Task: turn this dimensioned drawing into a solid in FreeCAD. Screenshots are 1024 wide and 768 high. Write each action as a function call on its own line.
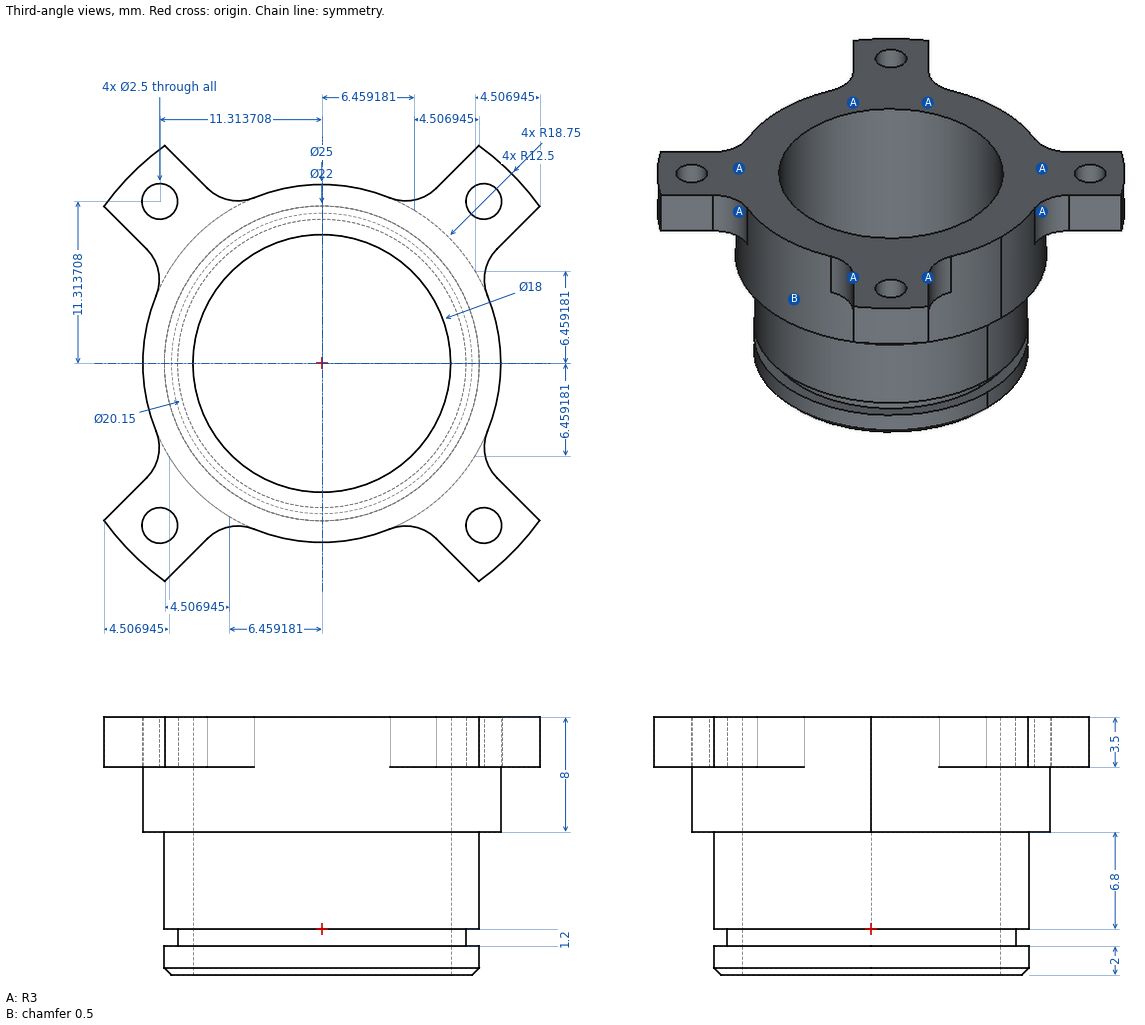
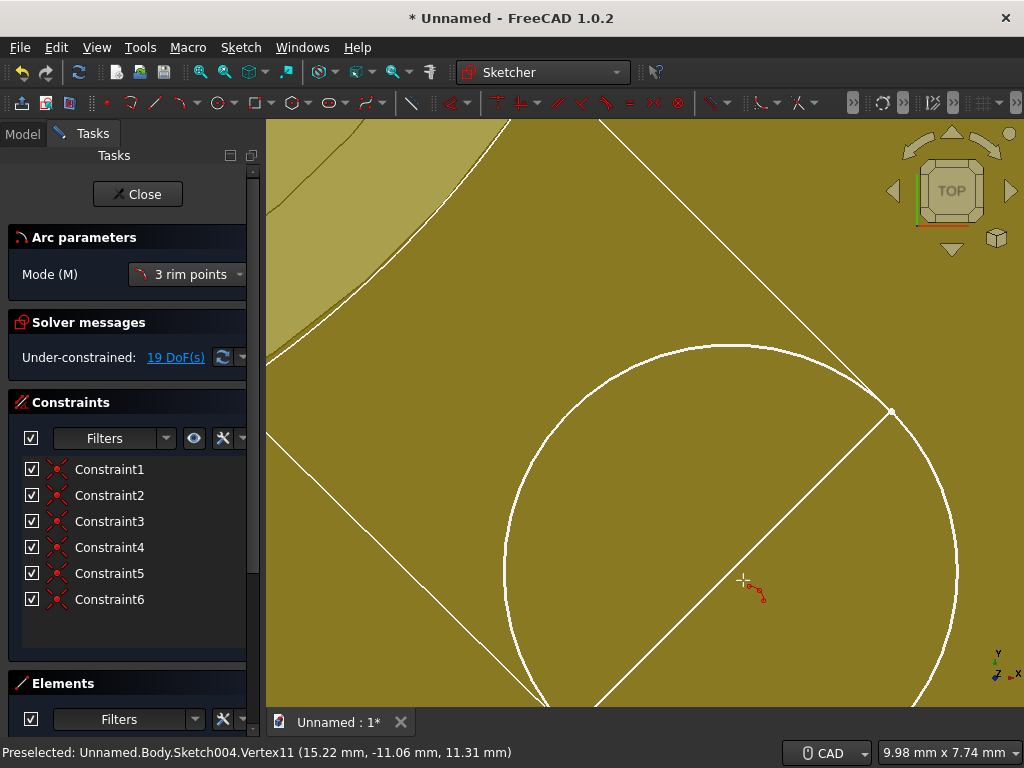
click(742, 578)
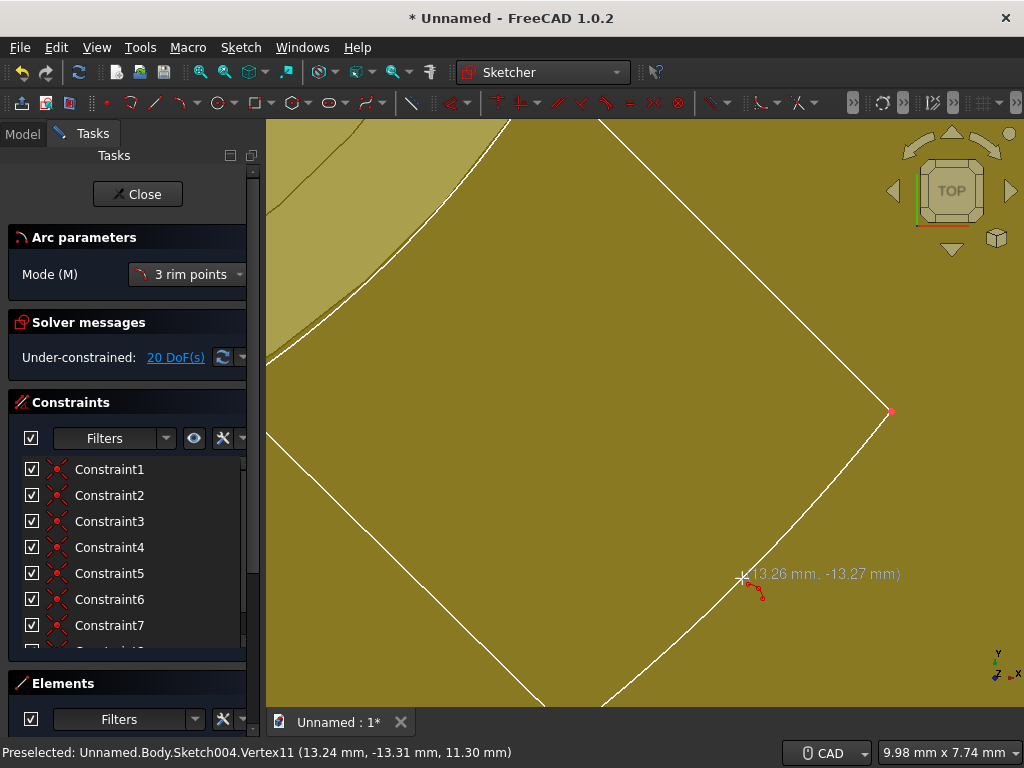
click(156, 104)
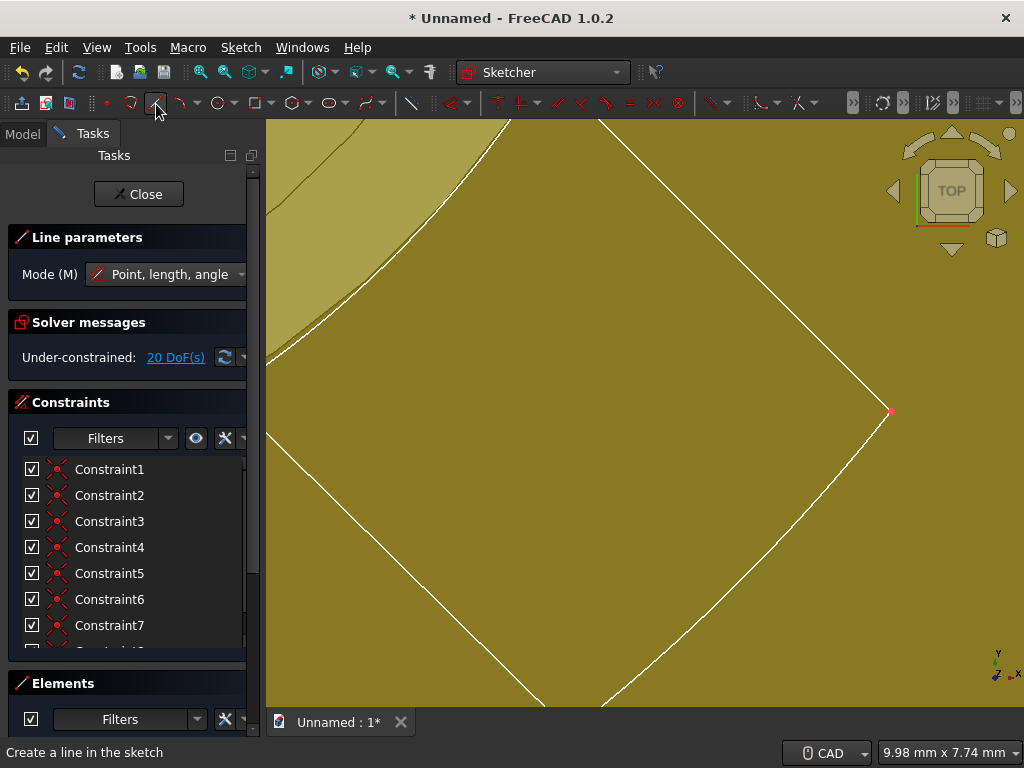
scroll(743, 580, down, 9)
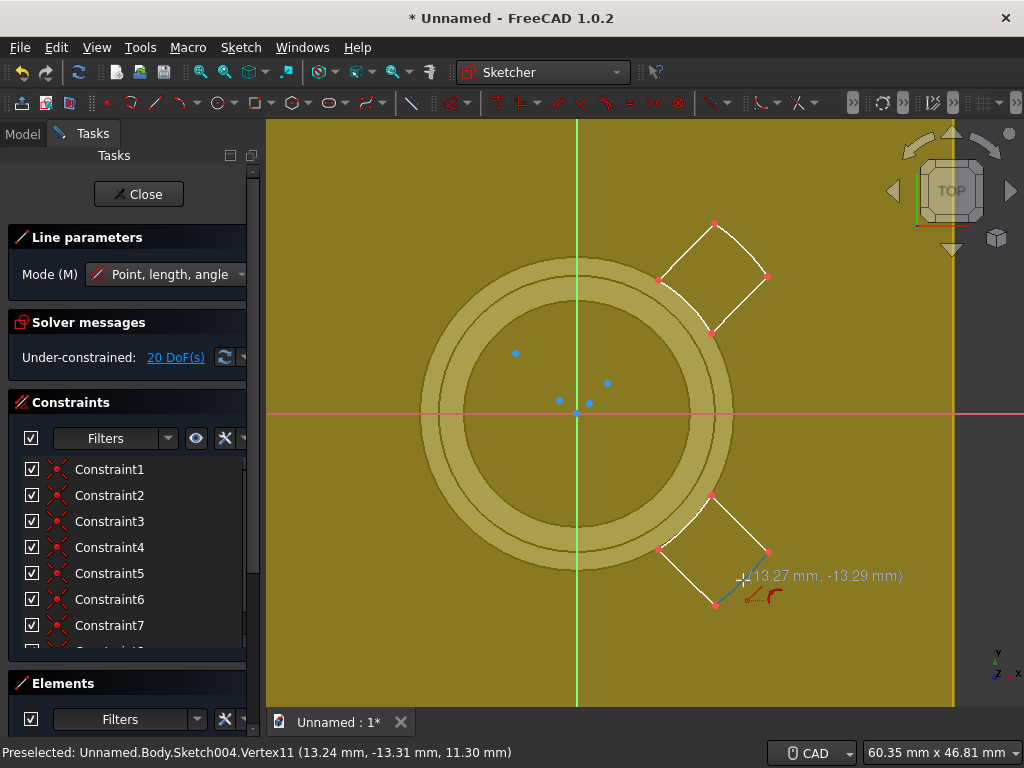
click(439, 605)
click(496, 548)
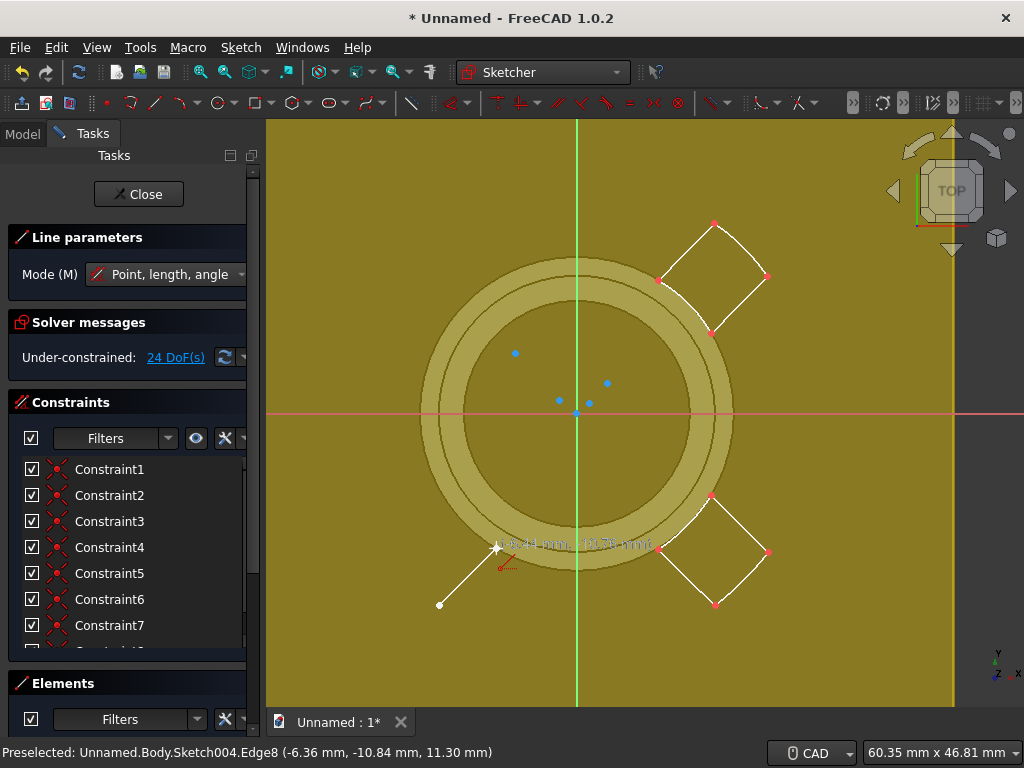
click(442, 495)
click(386, 552)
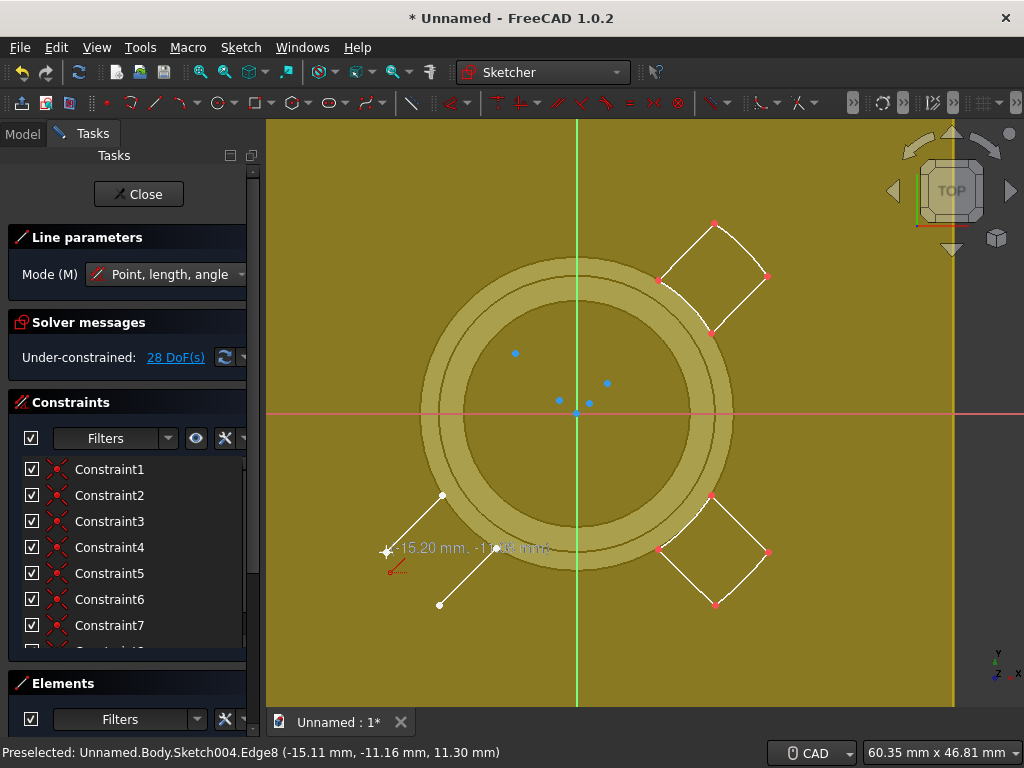
click(180, 104)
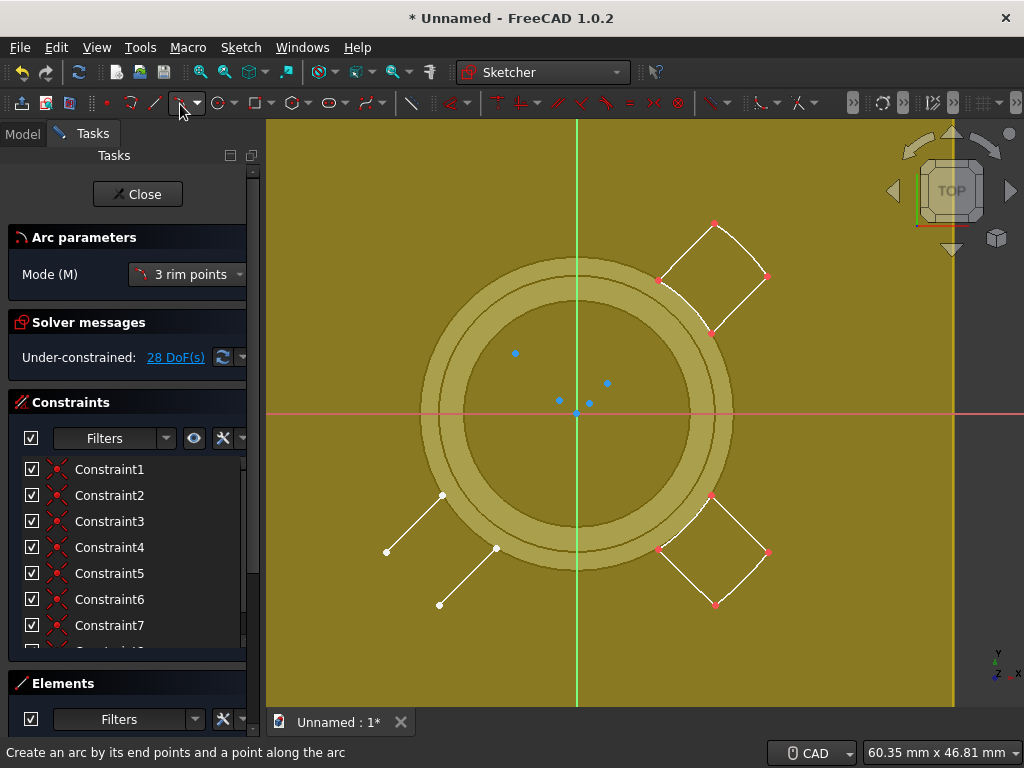
click(496, 549)
click(442, 496)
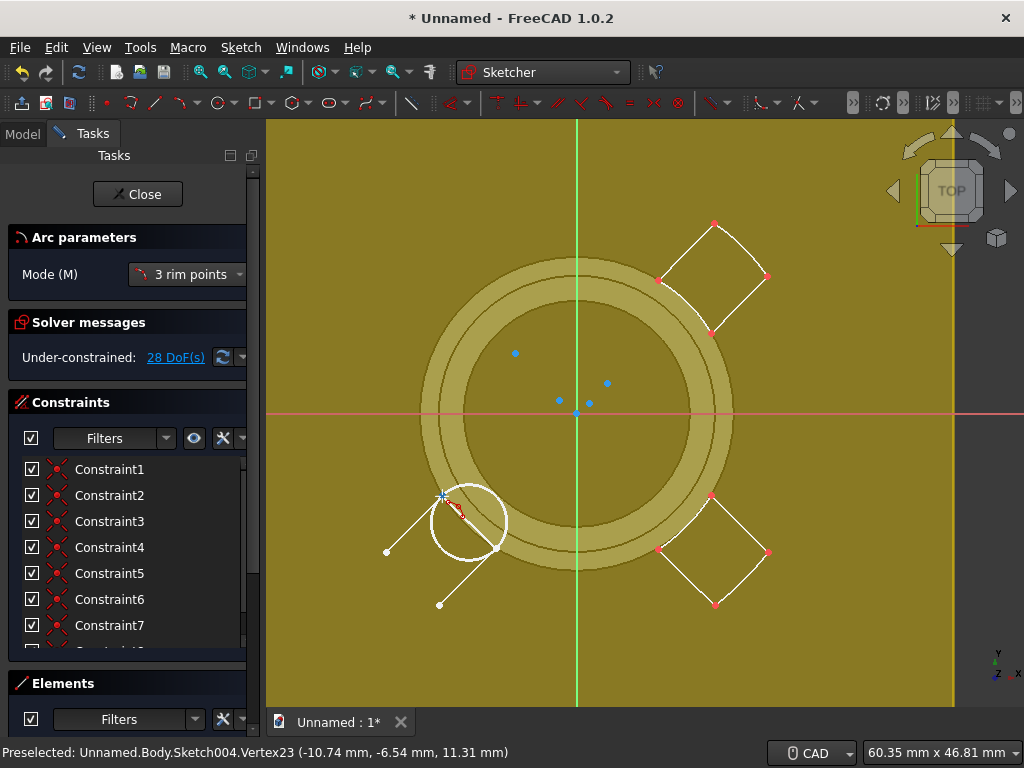
scroll(466, 525, up, 7)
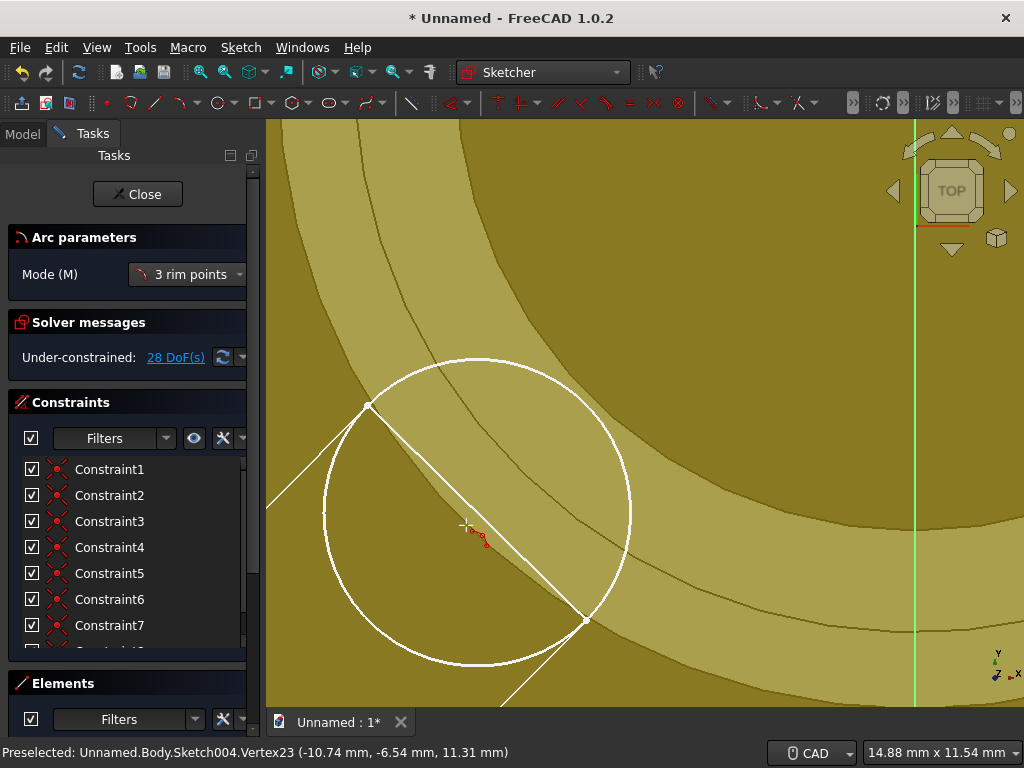
click(465, 522)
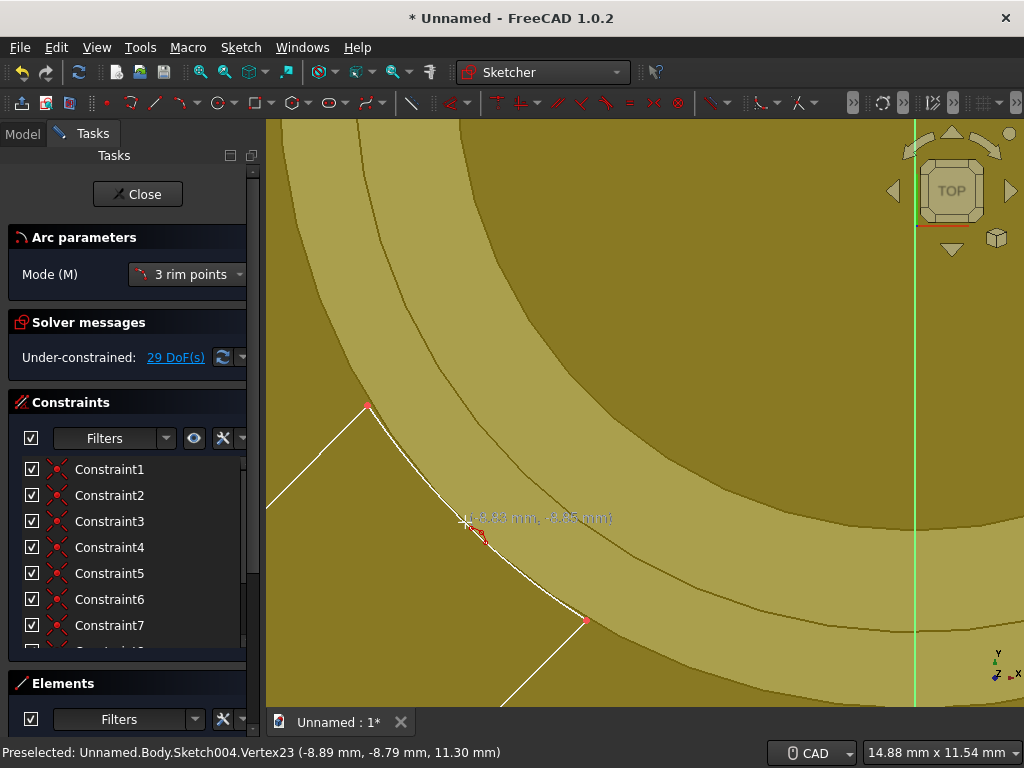
scroll(466, 525, down, 7)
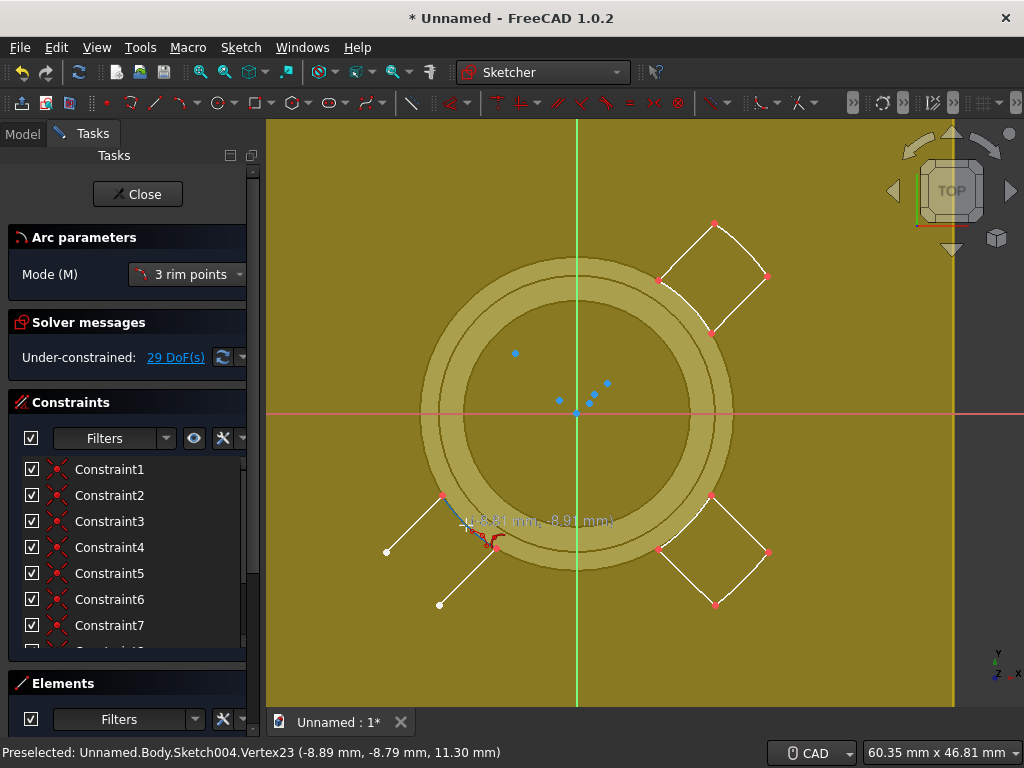
click(386, 553)
click(439, 606)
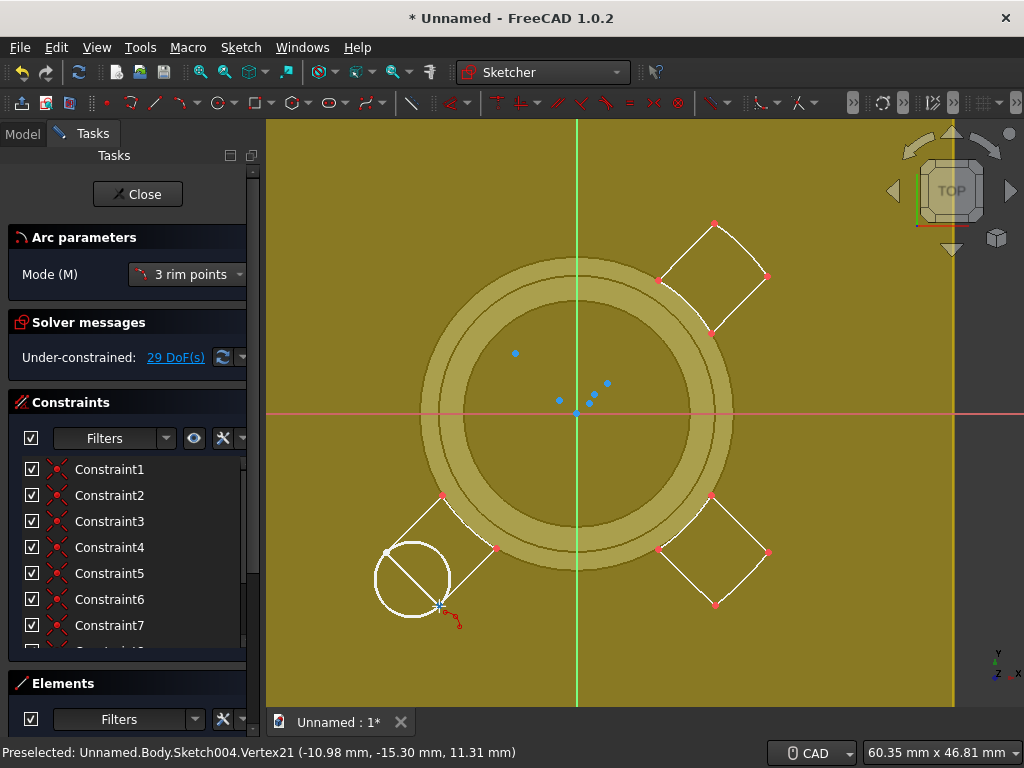
scroll(410, 580, up, 9)